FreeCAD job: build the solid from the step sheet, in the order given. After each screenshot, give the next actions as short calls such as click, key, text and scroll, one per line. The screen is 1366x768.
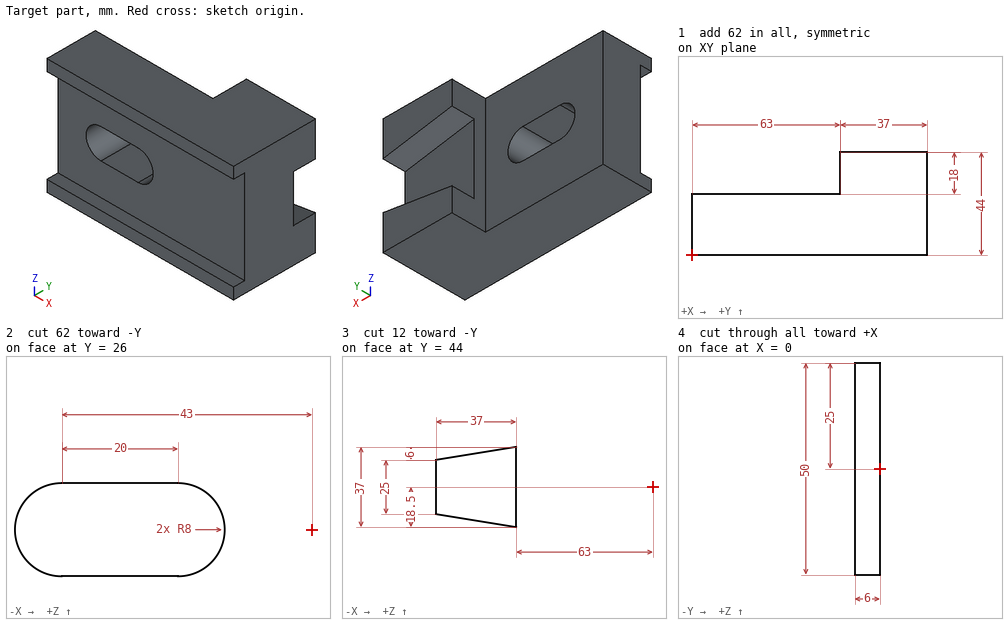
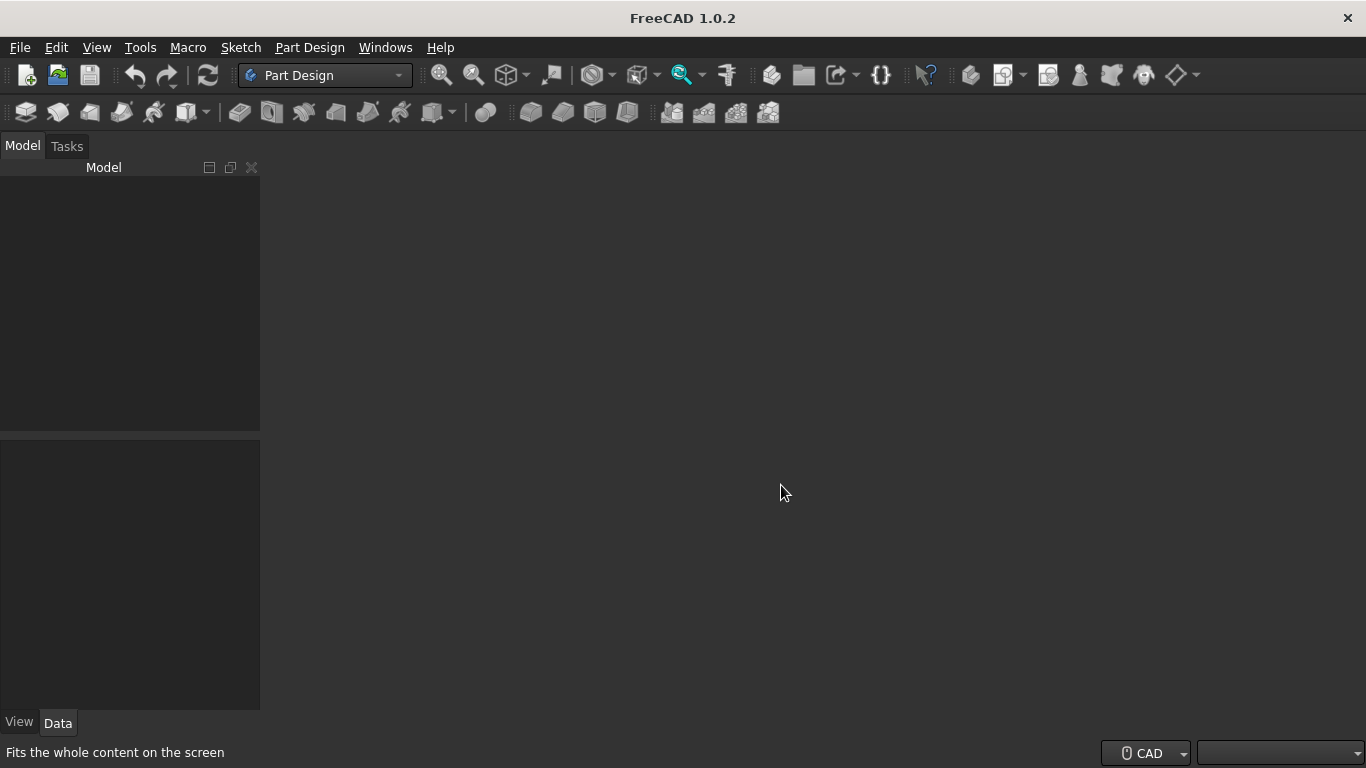
click(26, 76)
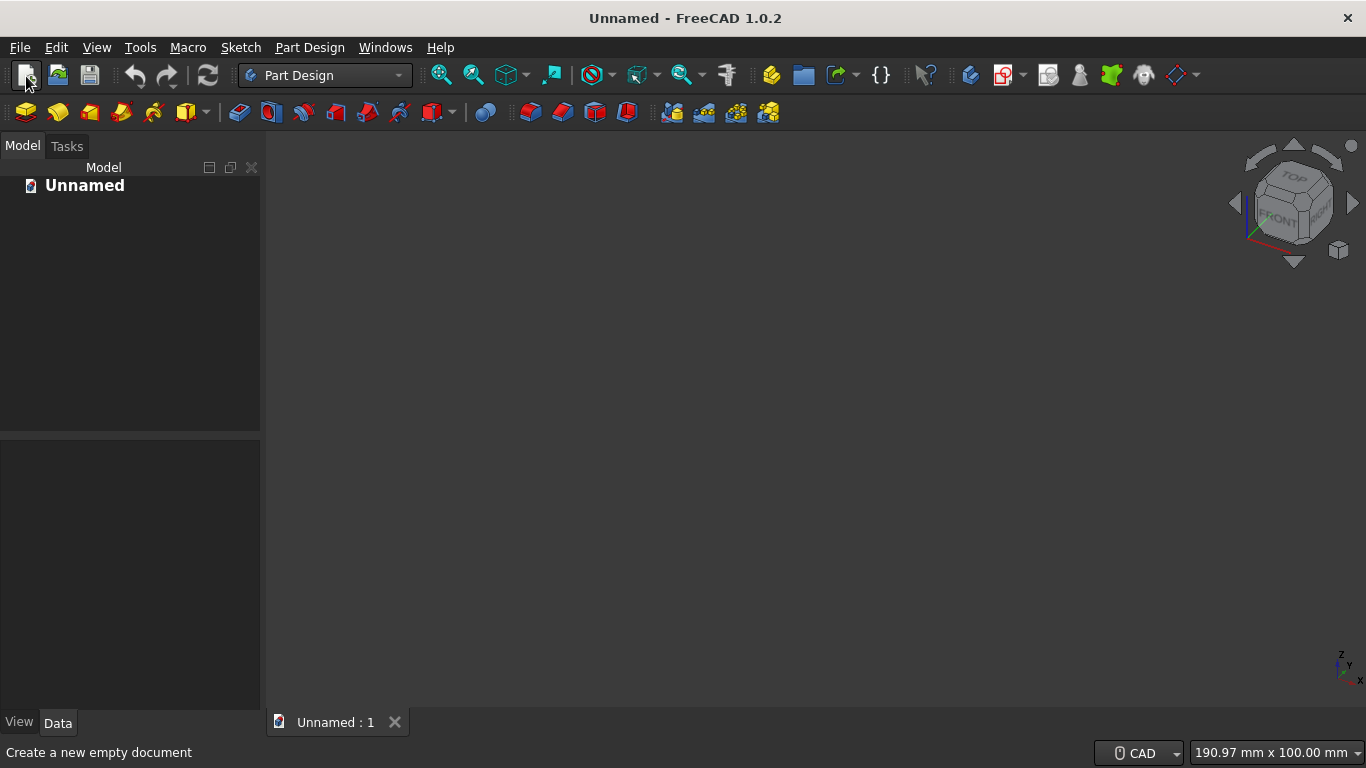
click(1004, 76)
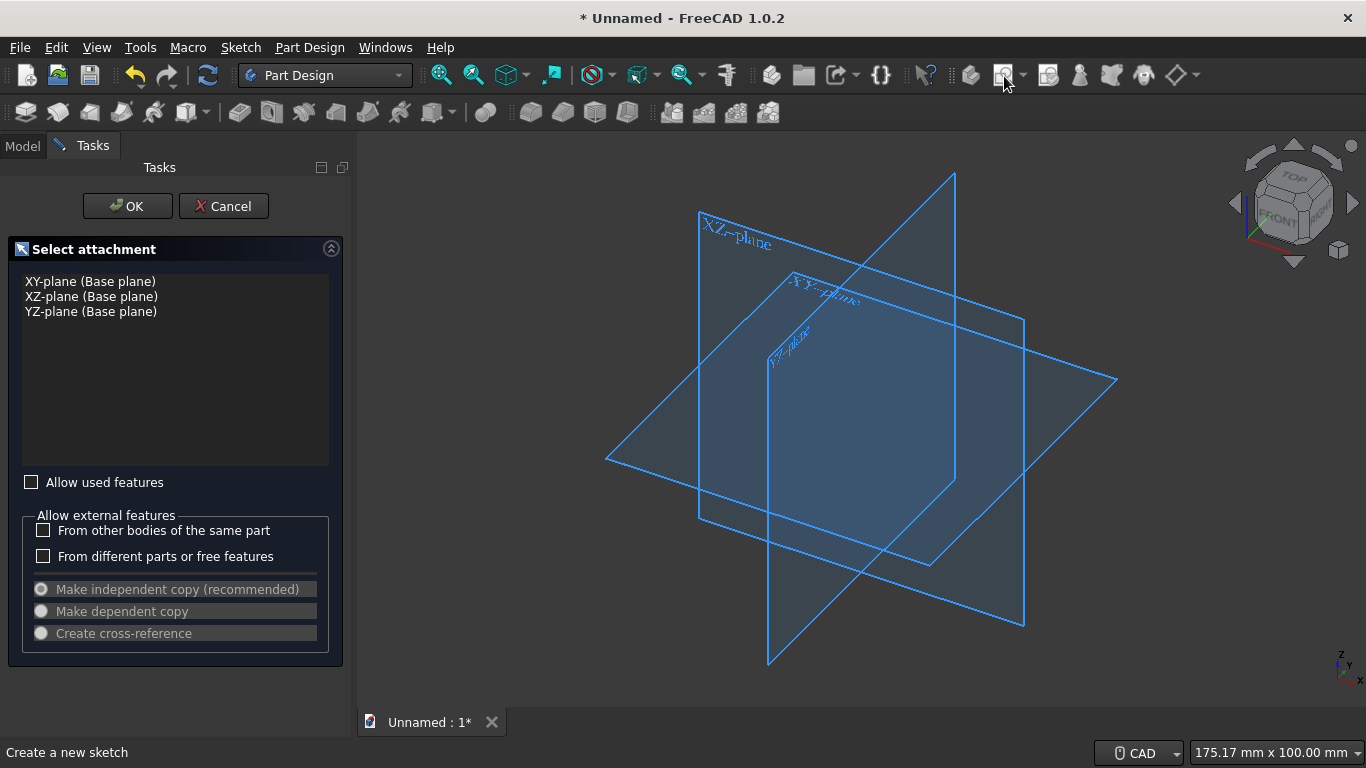
click(82, 282)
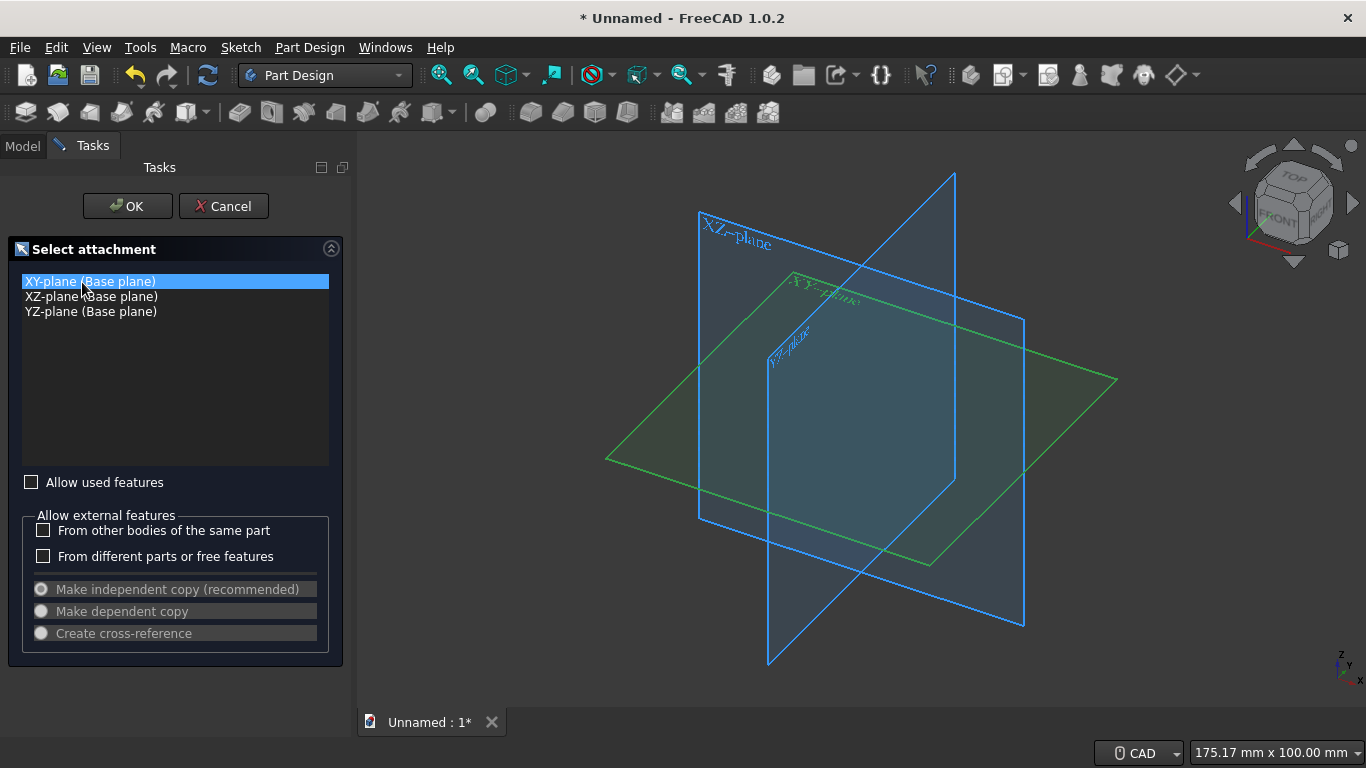
click(128, 206)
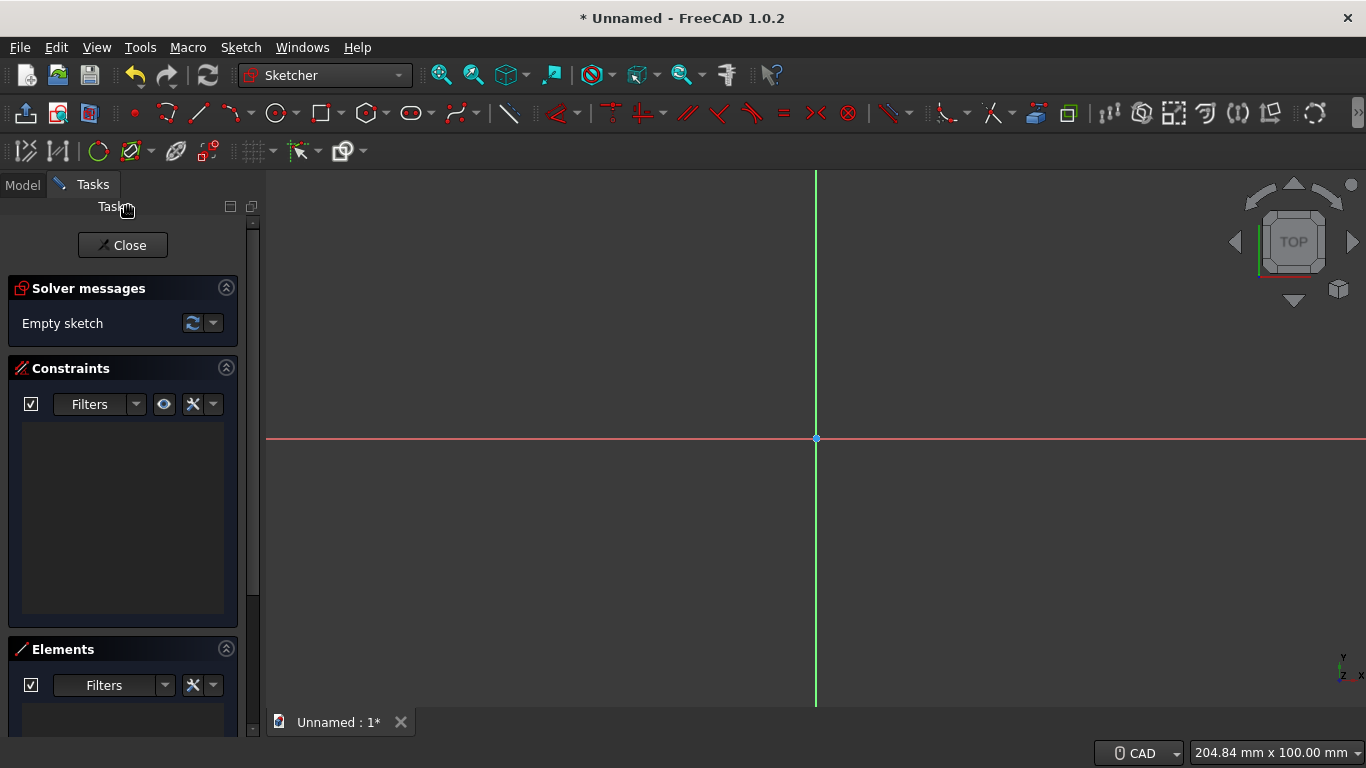
scroll(294, 679, down, 1)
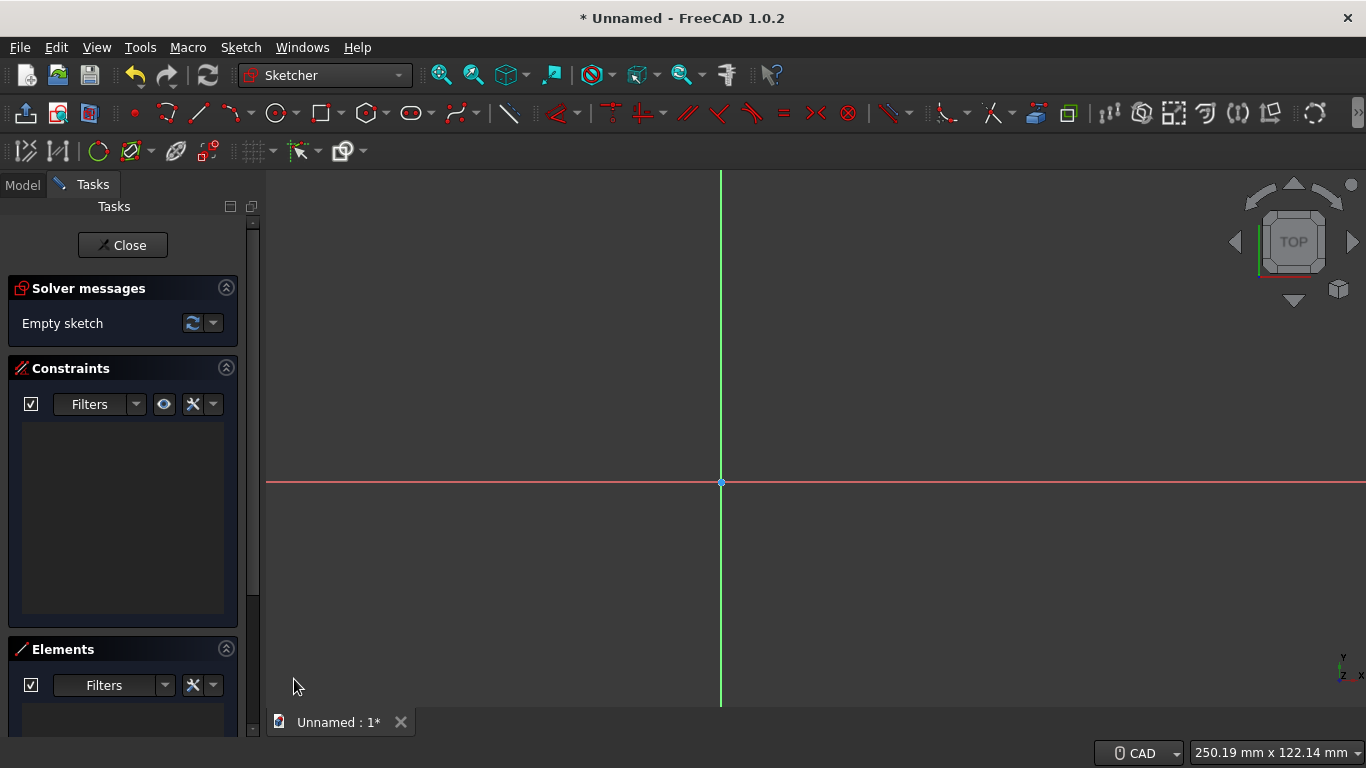
scroll(1201, 278, up, 2)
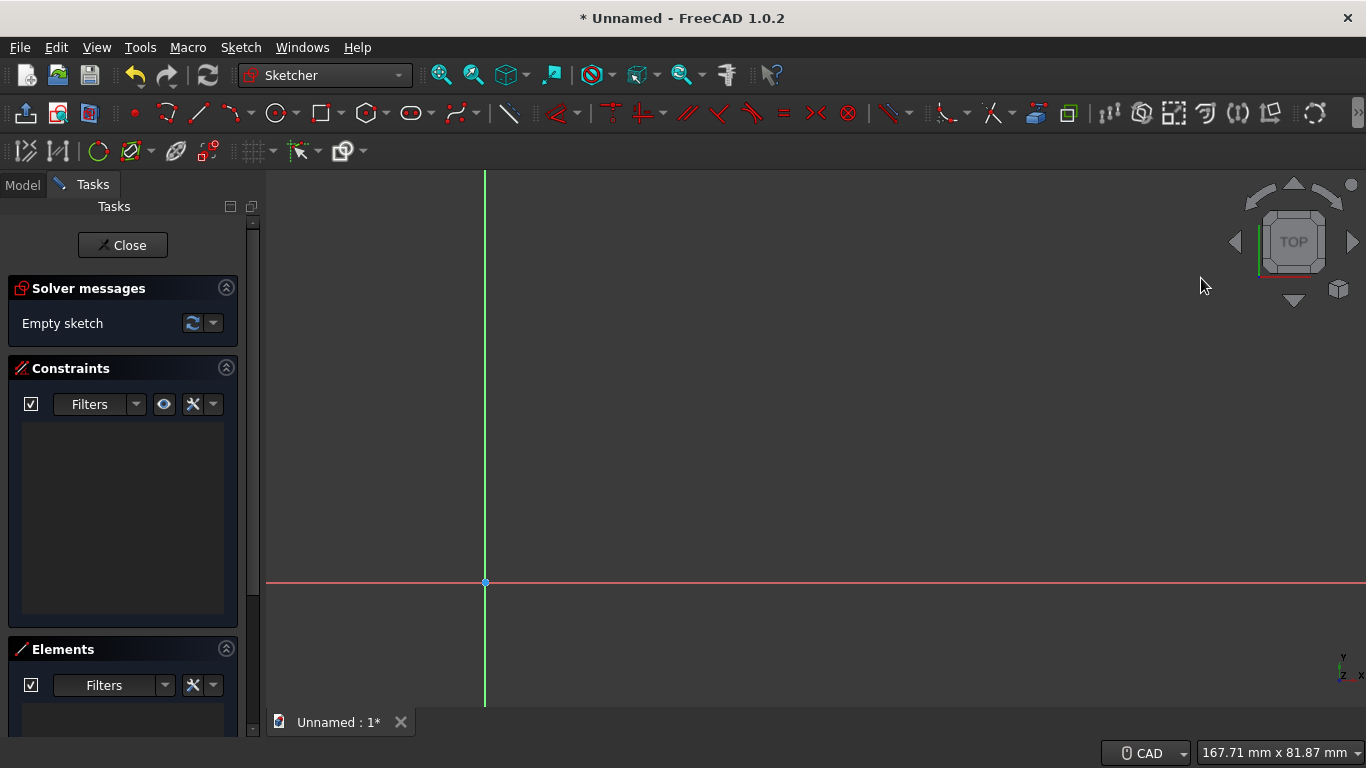
click(168, 114)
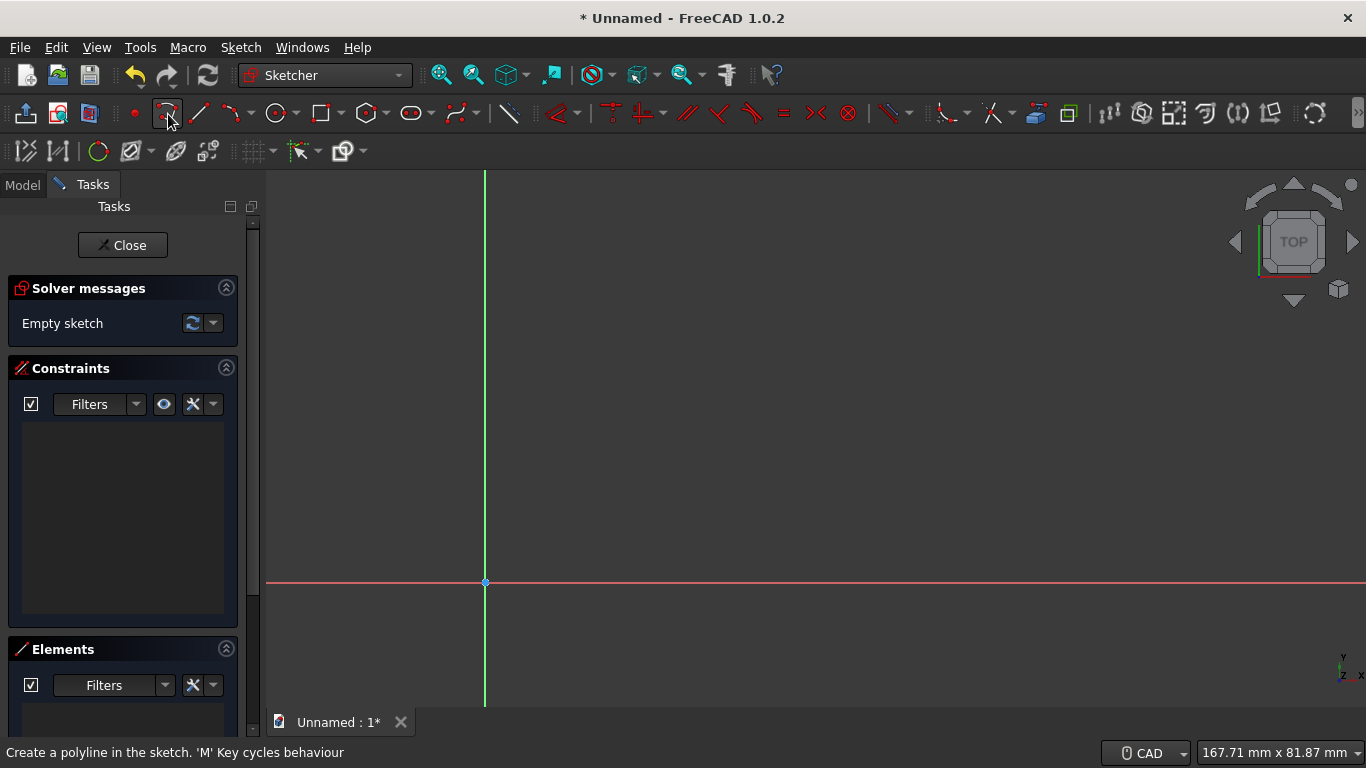
click(485, 583)
click(1141, 574)
click(1141, 294)
click(898, 294)
click(898, 412)
click(494, 412)
click(485, 583)
key(Escape)
key(Escape)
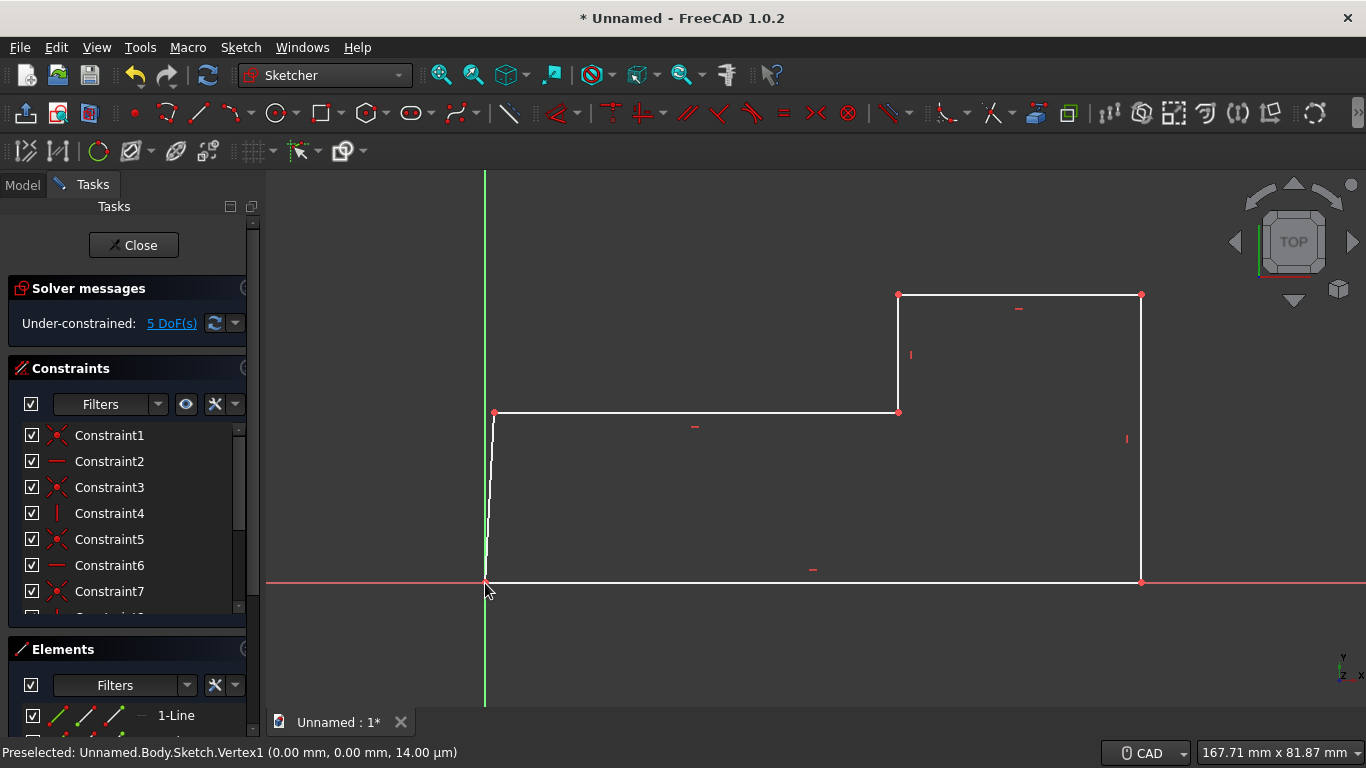
click(488, 532)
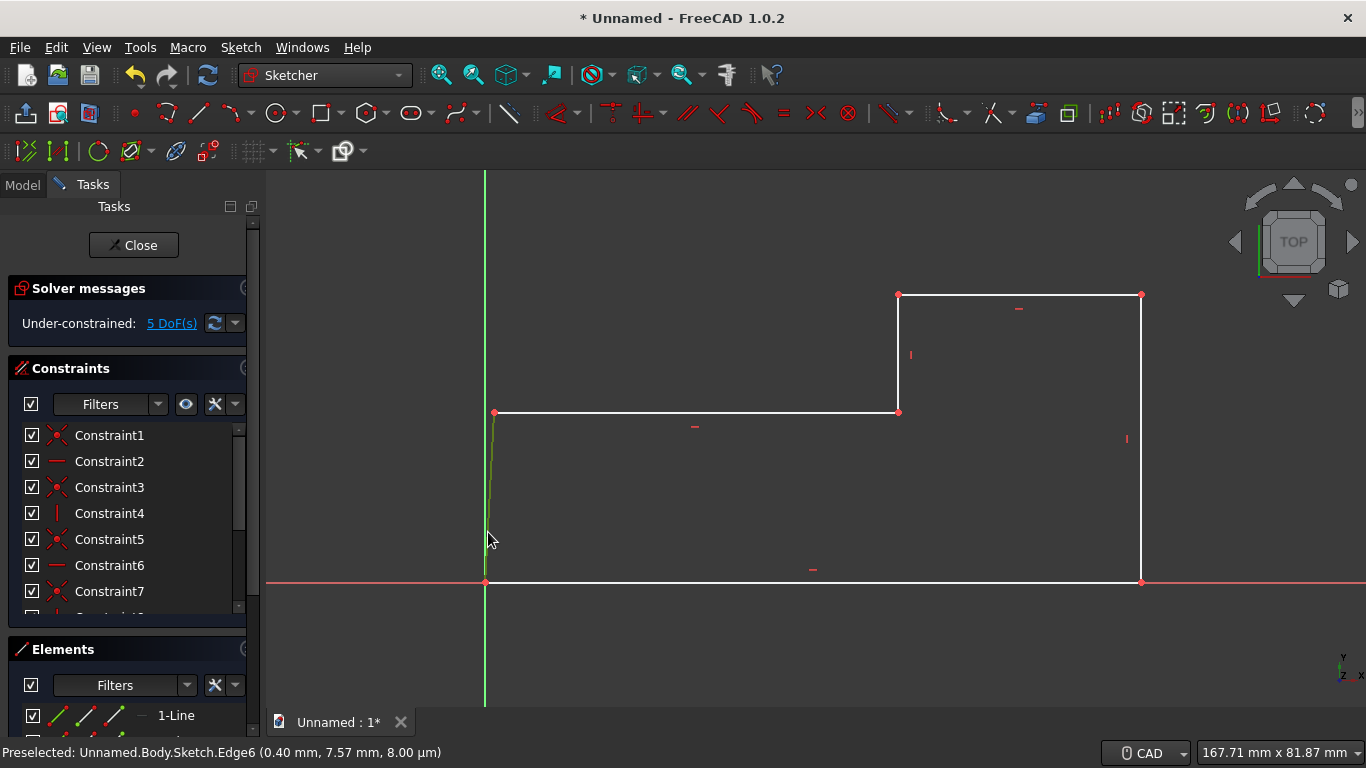
click(666, 114)